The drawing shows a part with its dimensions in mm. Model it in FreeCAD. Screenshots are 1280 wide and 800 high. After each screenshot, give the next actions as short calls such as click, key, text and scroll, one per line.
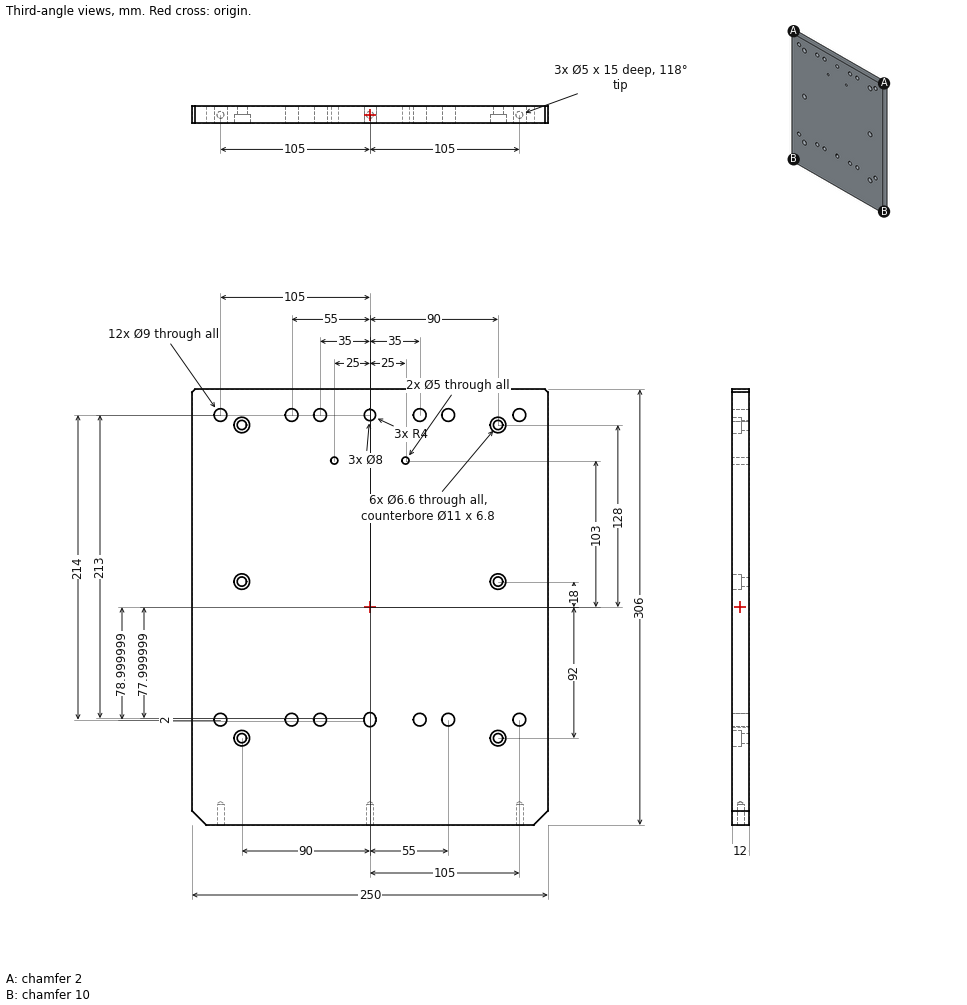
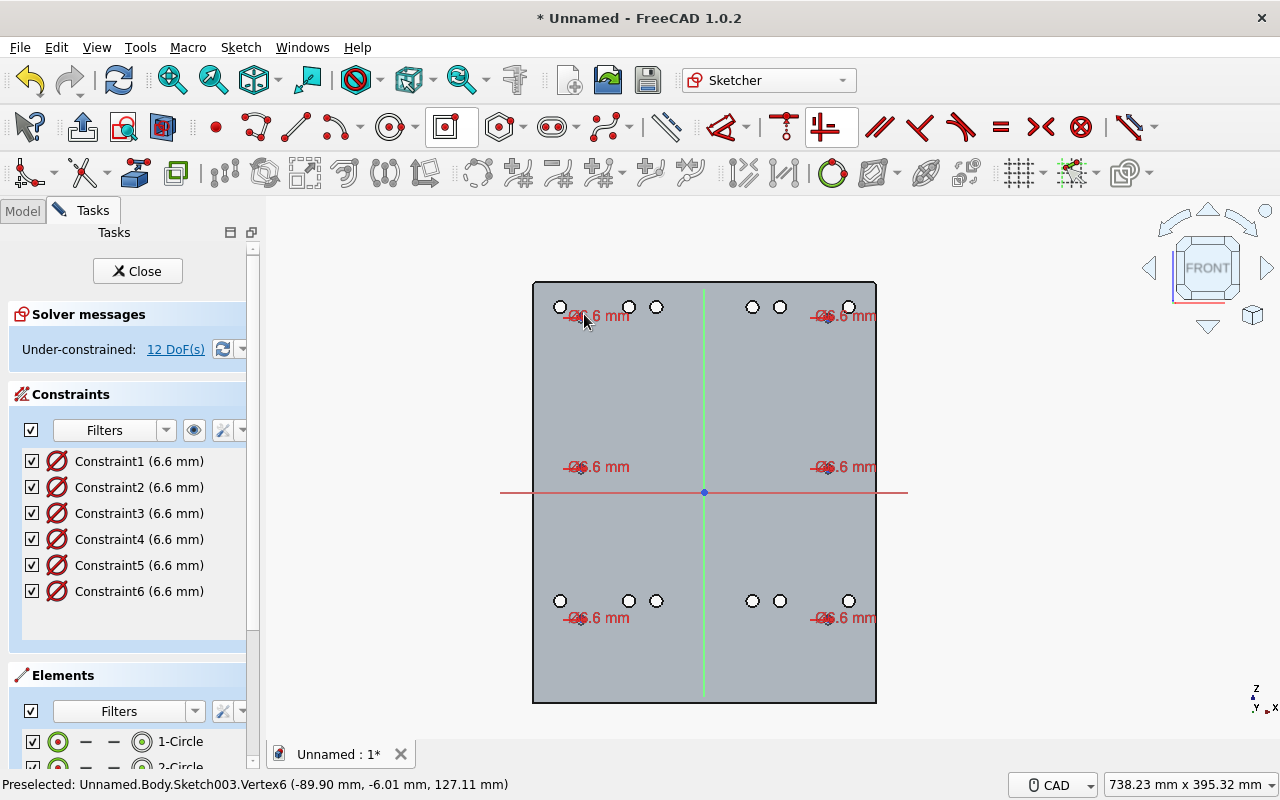
click(828, 318)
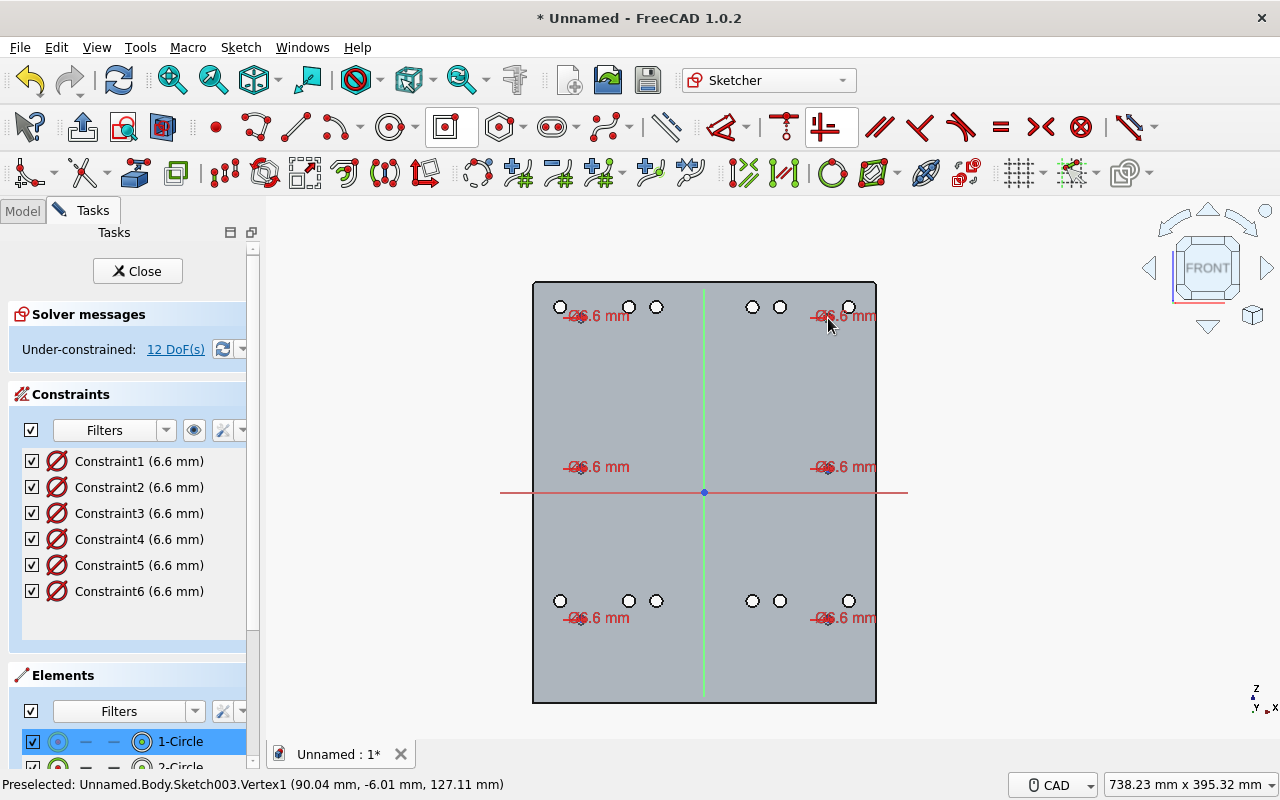
click(828, 469)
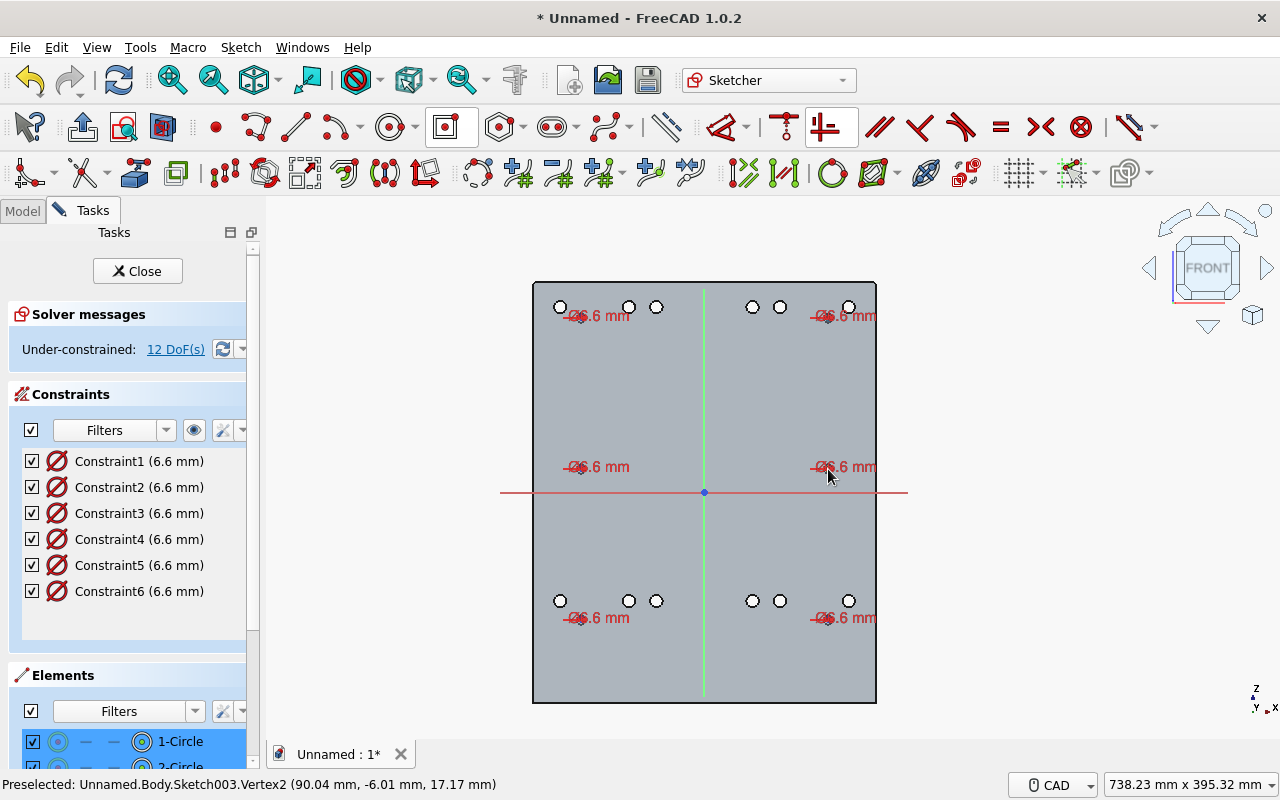
click(852, 128)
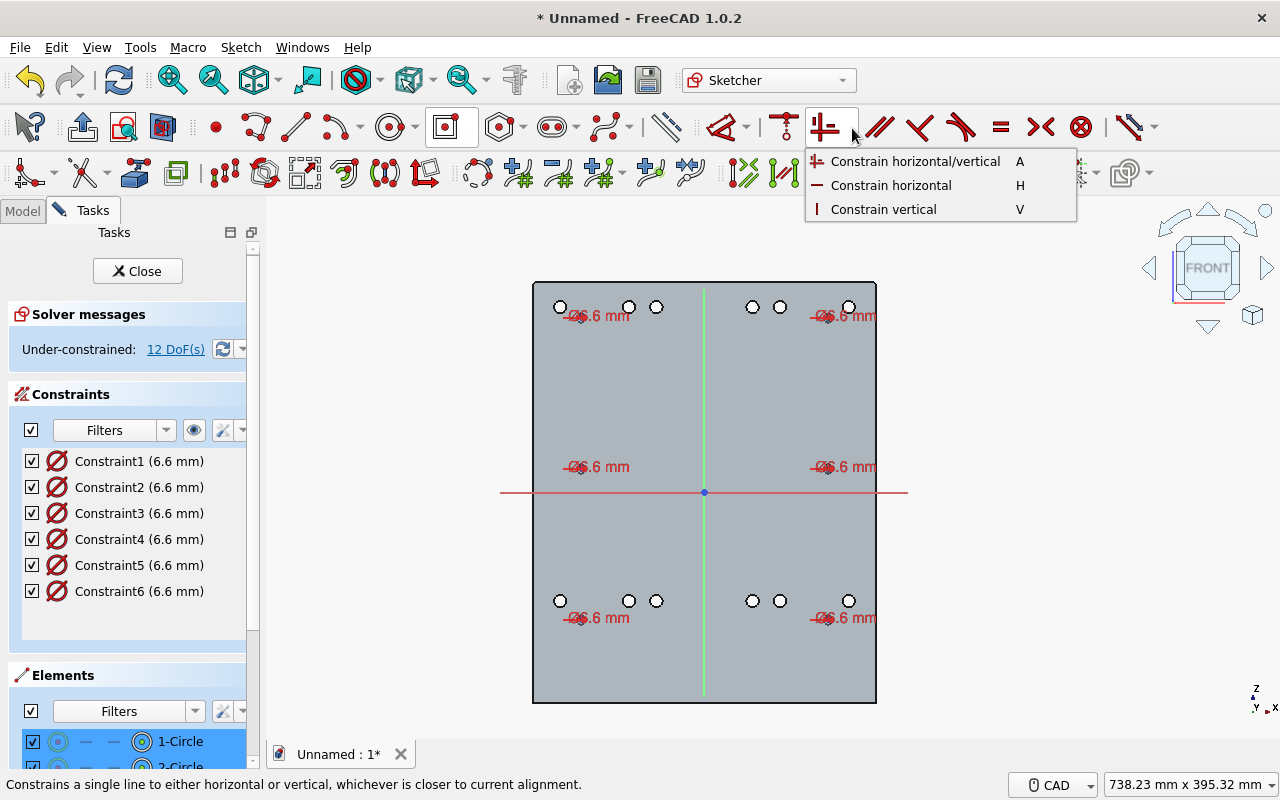
click(941, 209)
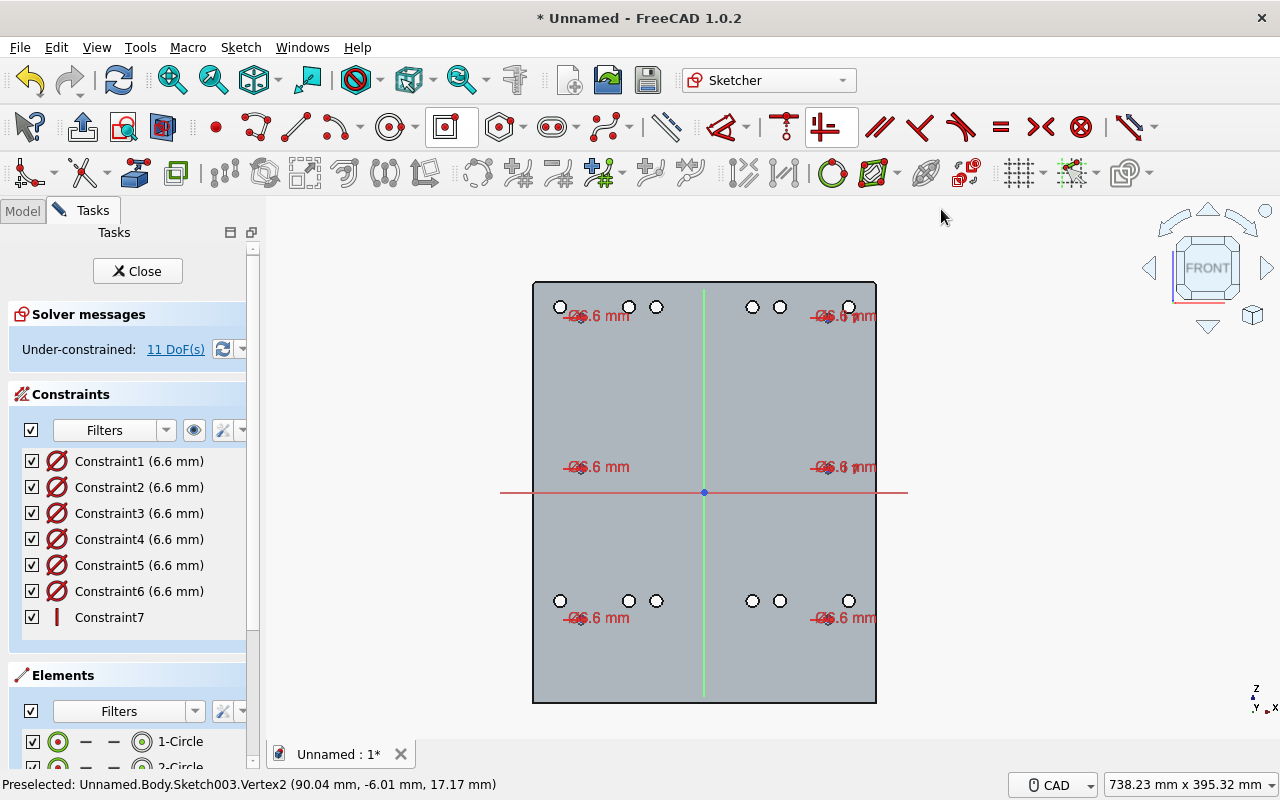
click(828, 469)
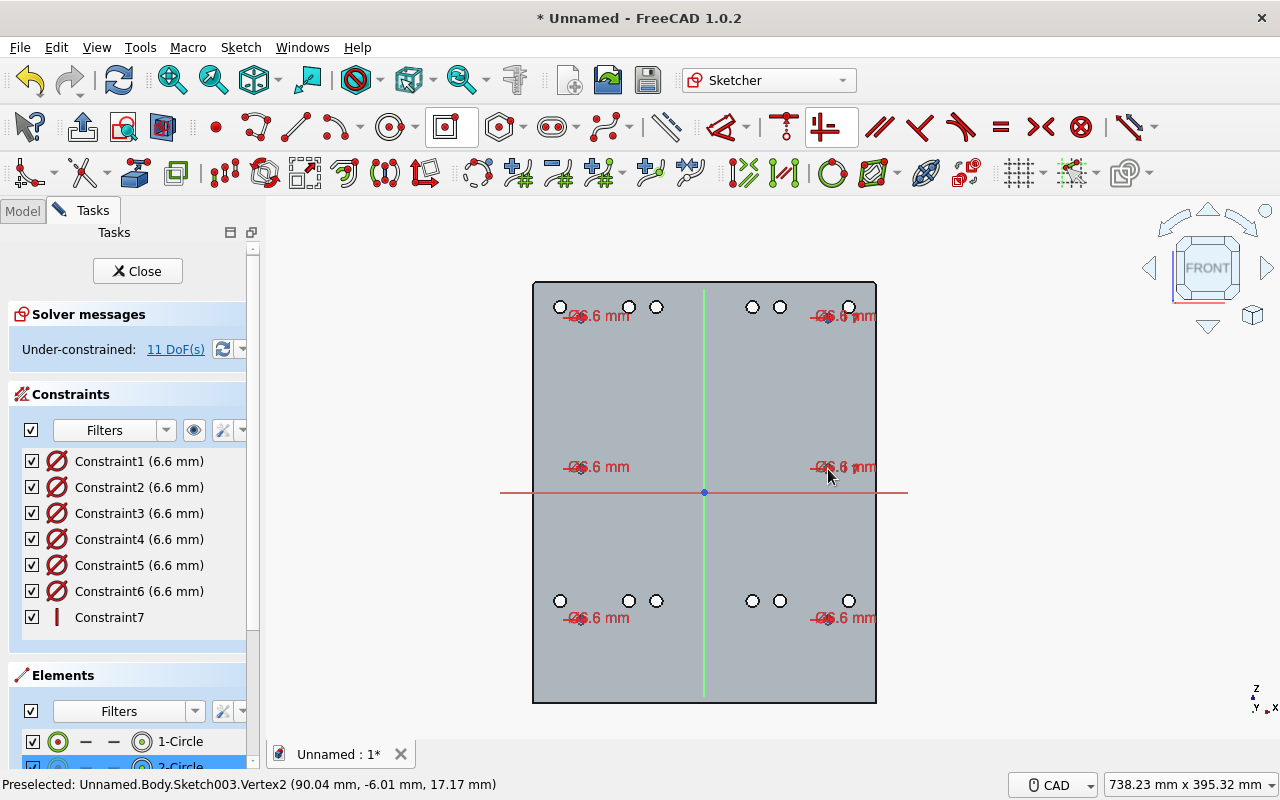
click(828, 620)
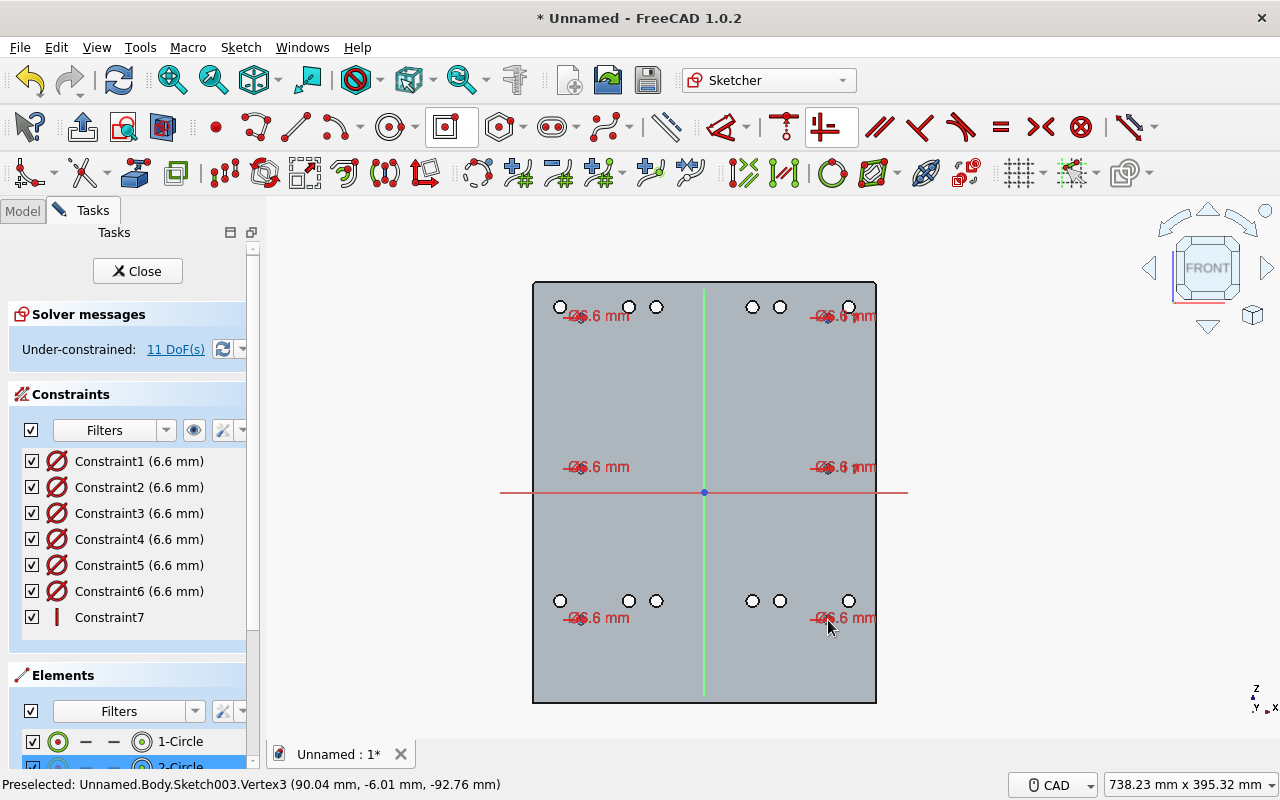
key(v)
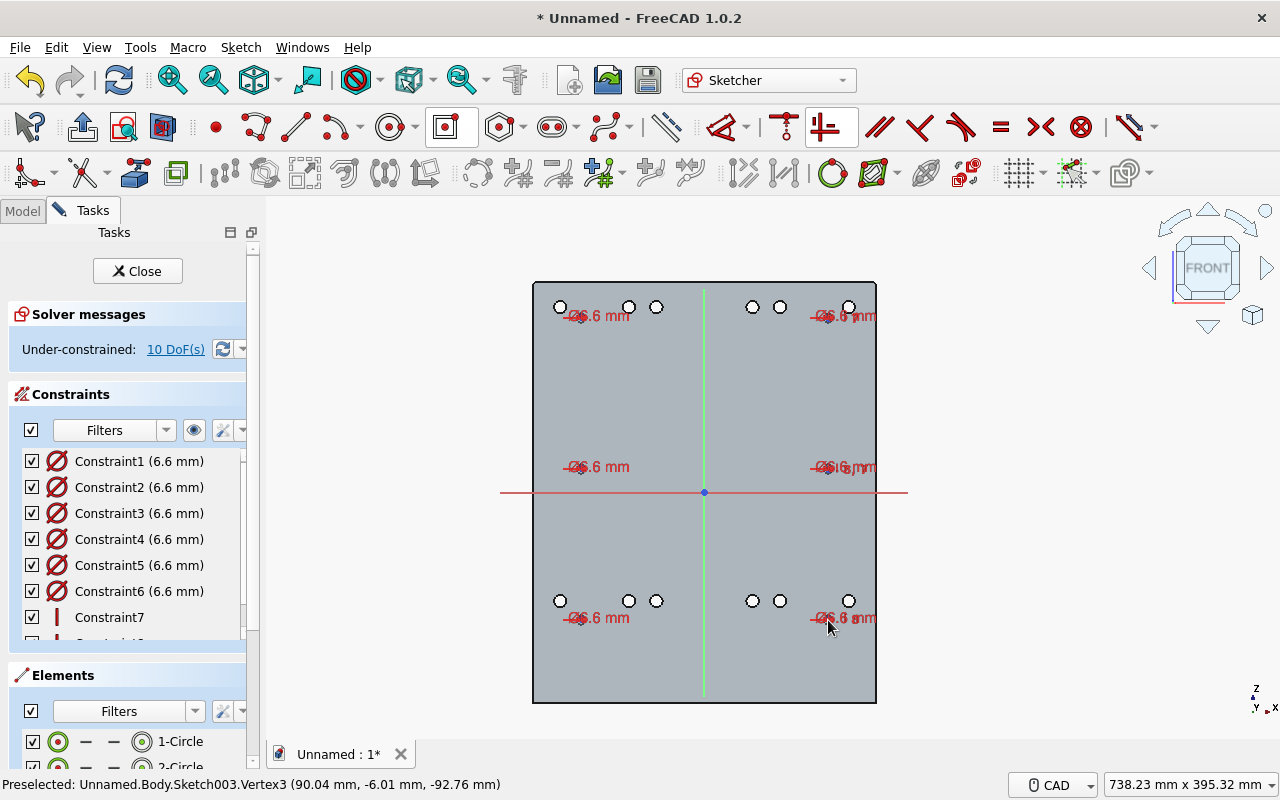
click(828, 620)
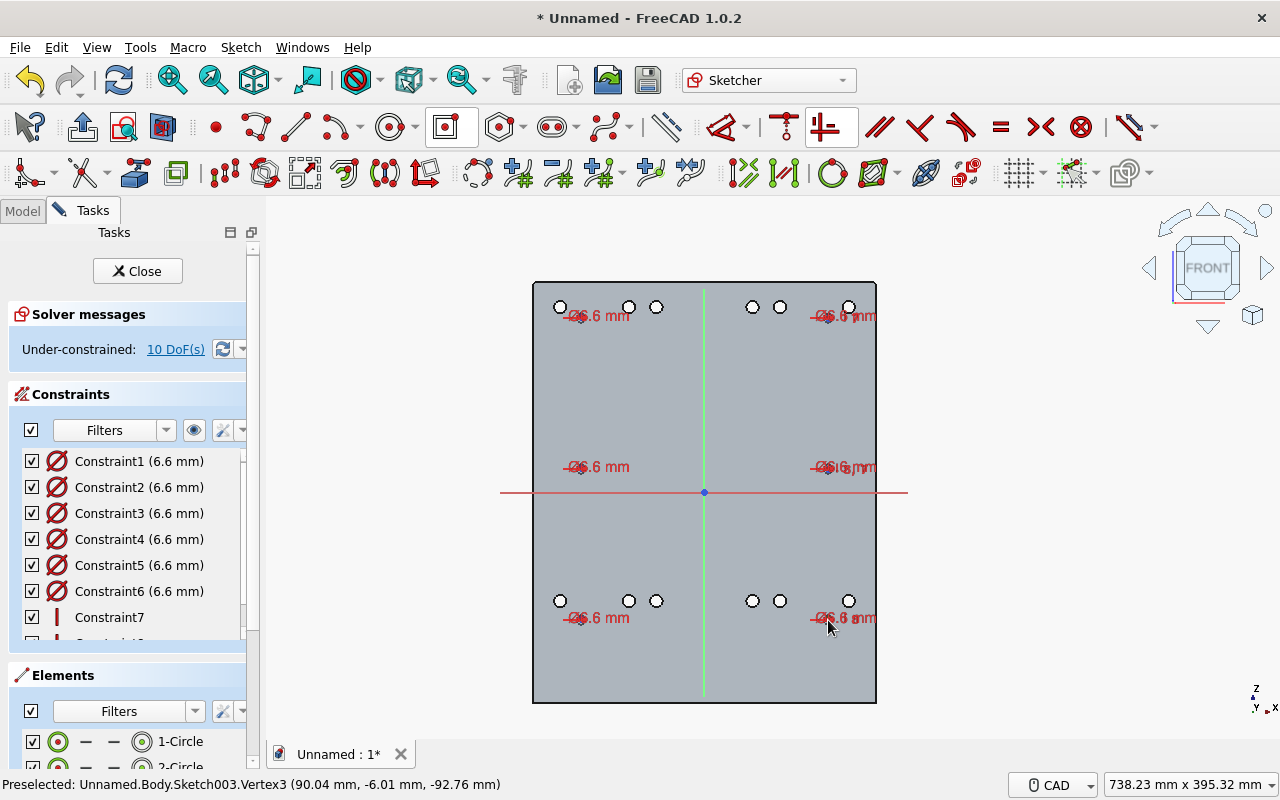
click(581, 620)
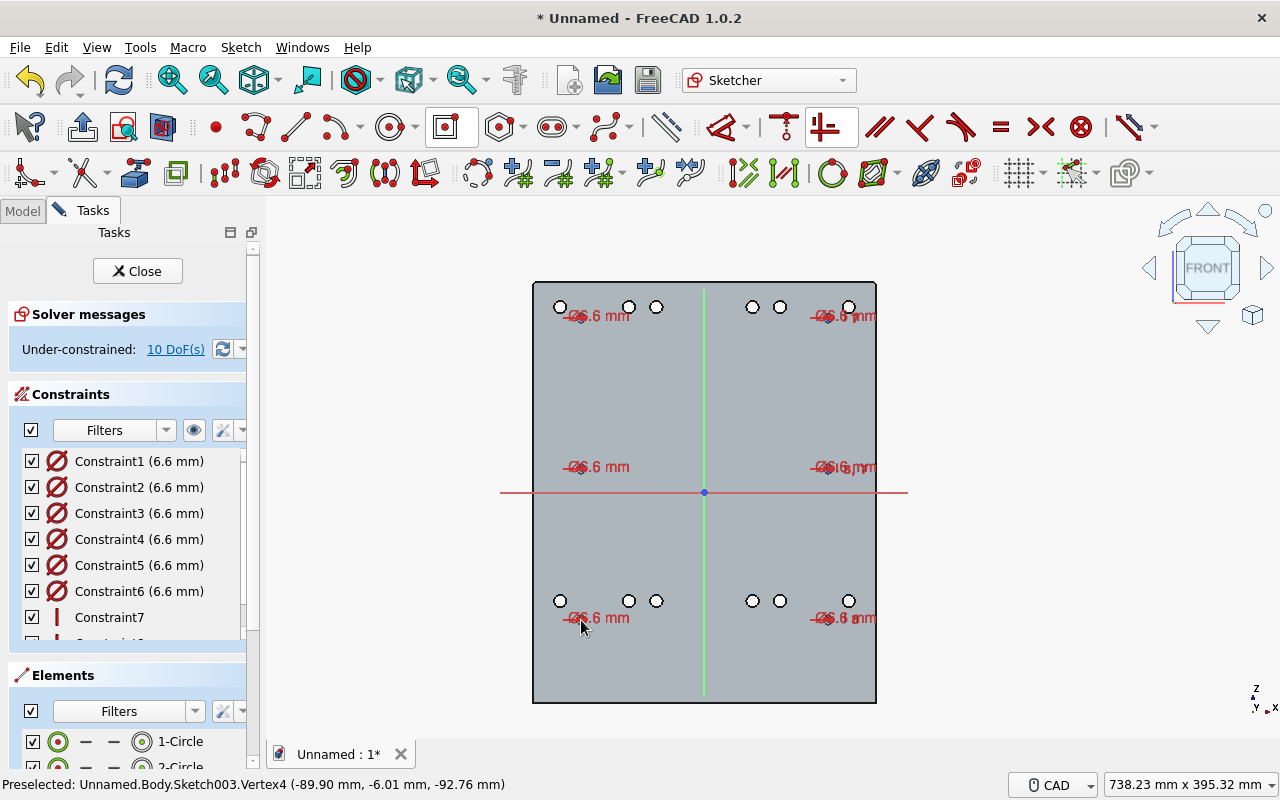
click(852, 128)